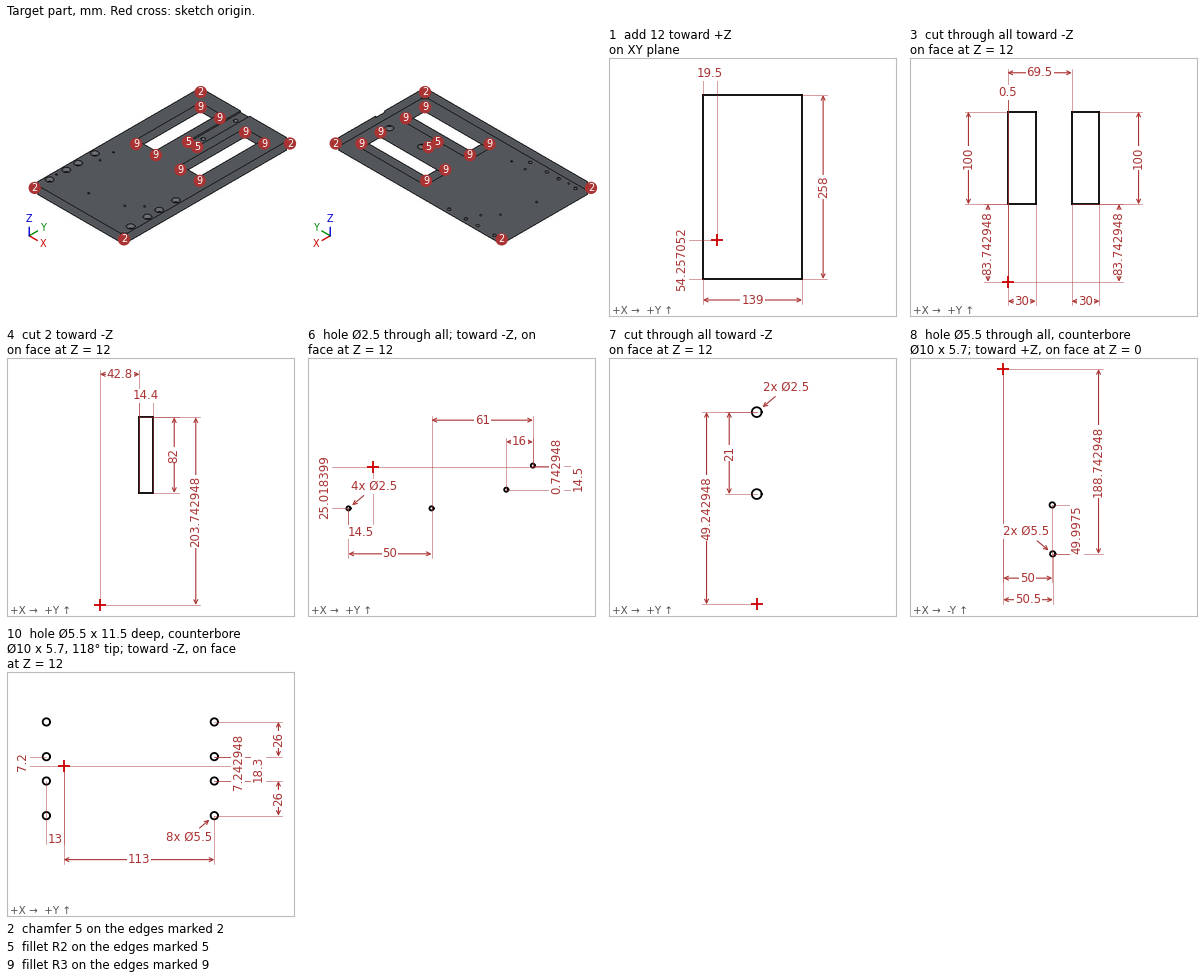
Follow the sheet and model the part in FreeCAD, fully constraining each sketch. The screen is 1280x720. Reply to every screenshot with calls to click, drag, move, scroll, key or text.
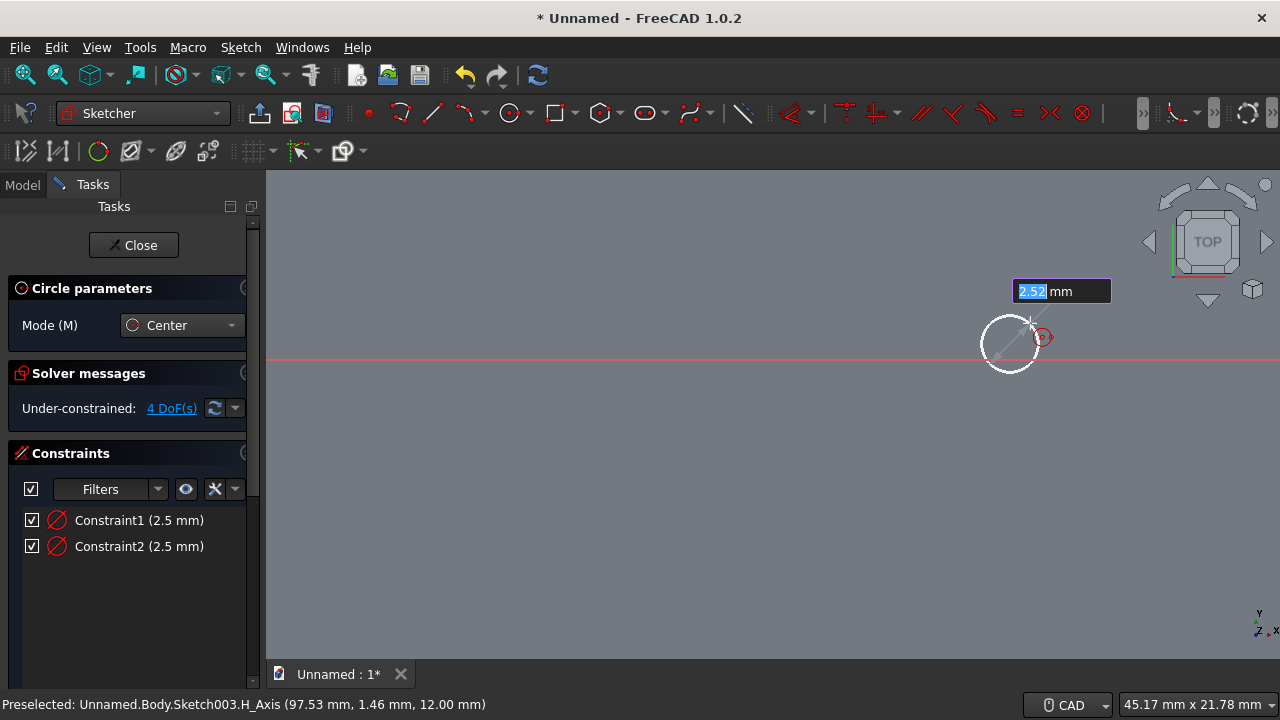
text(2.5)
key(Return)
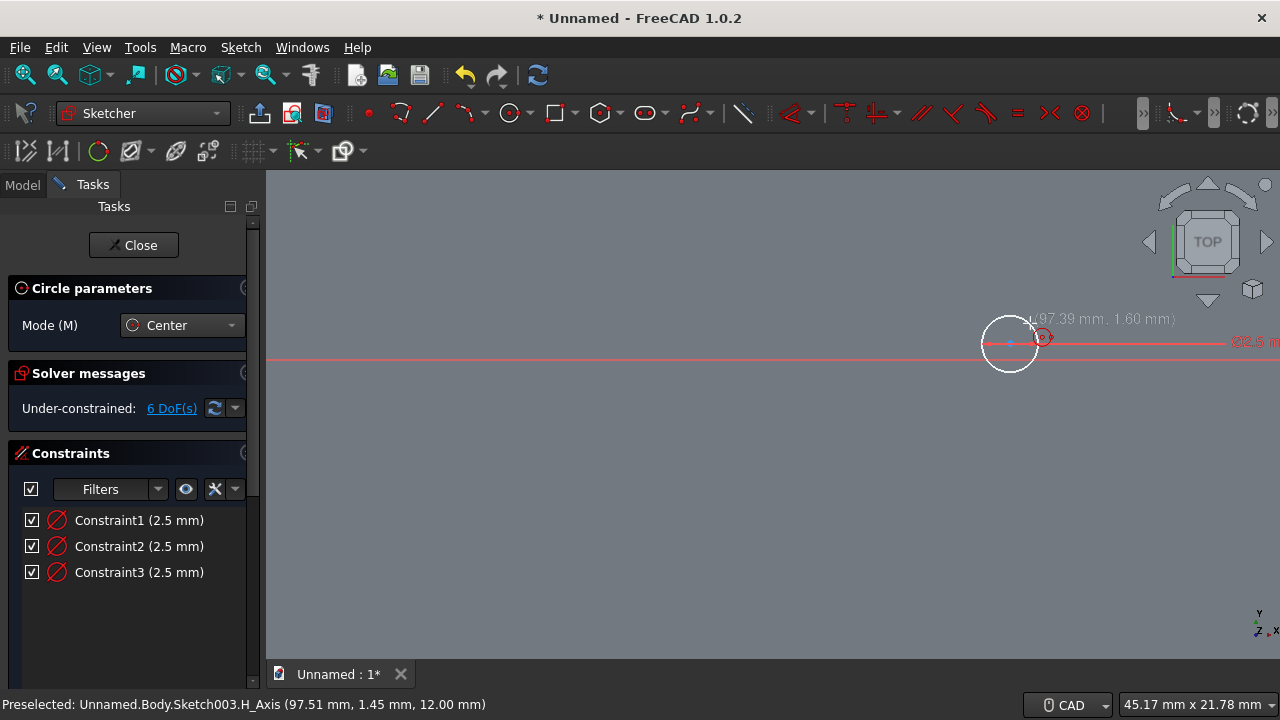
scroll(1012, 343, down, 7)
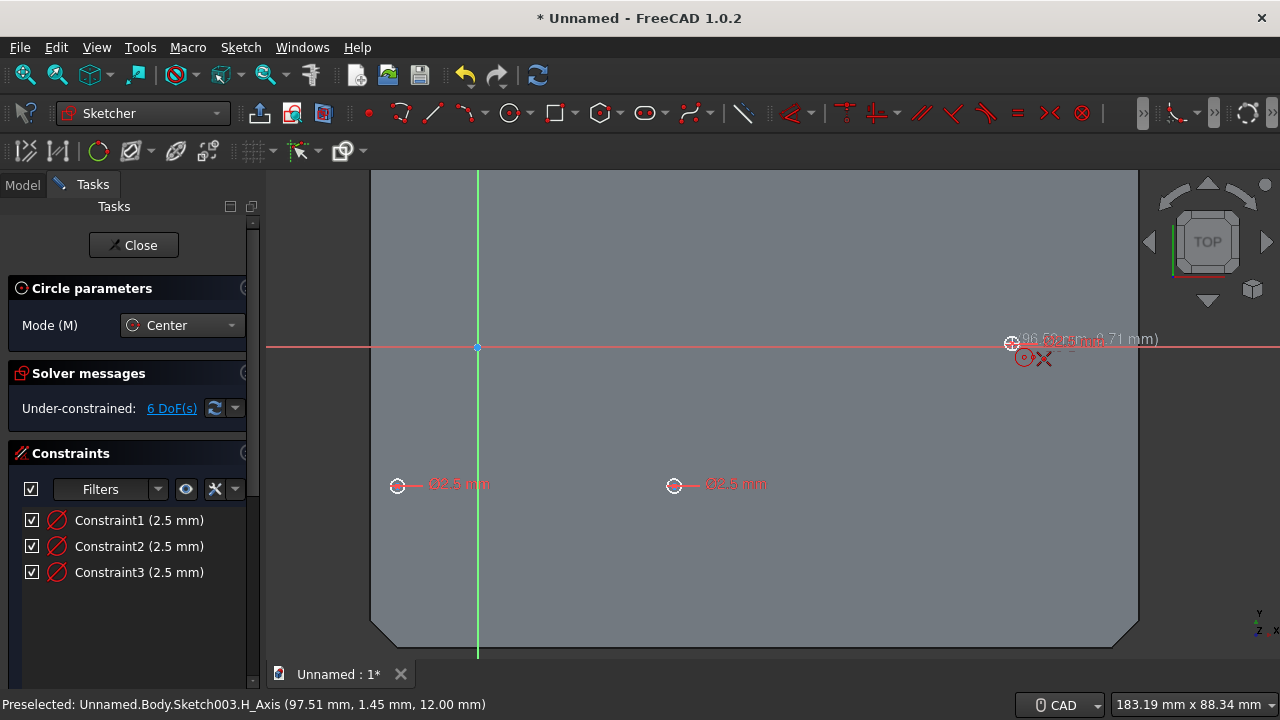
scroll(923, 424, up, 6)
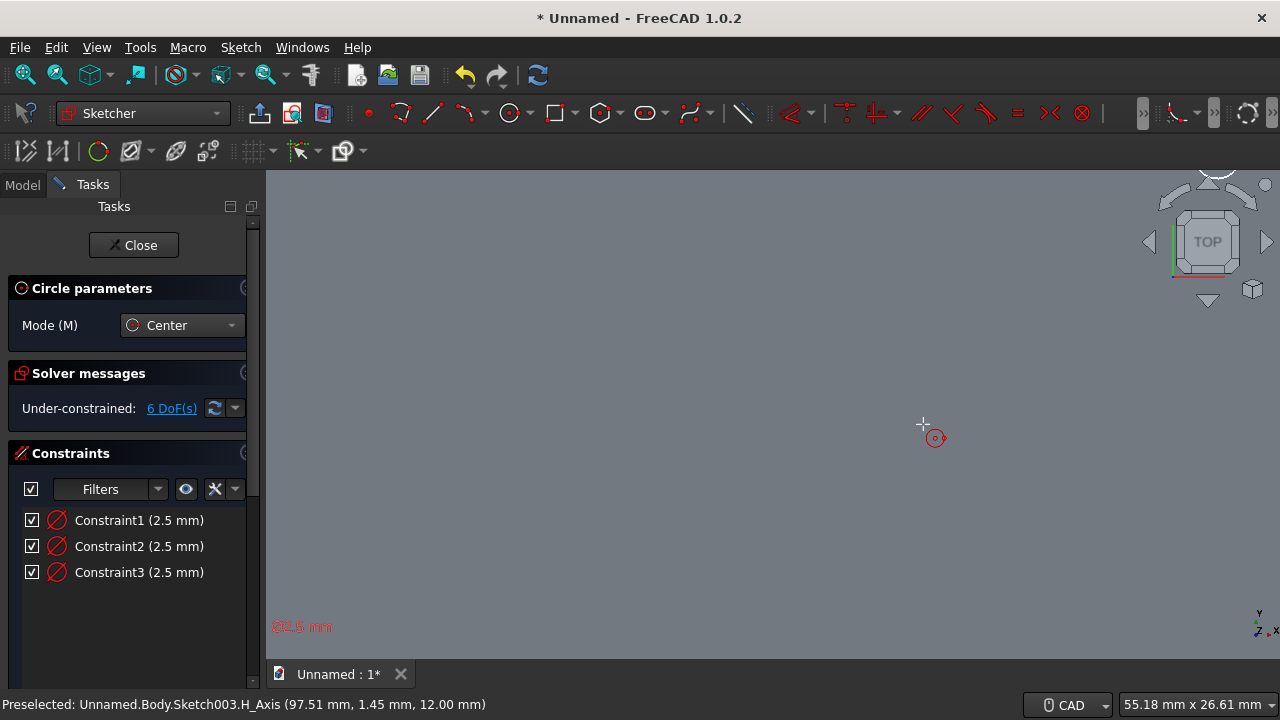
click(923, 421)
move(939, 405)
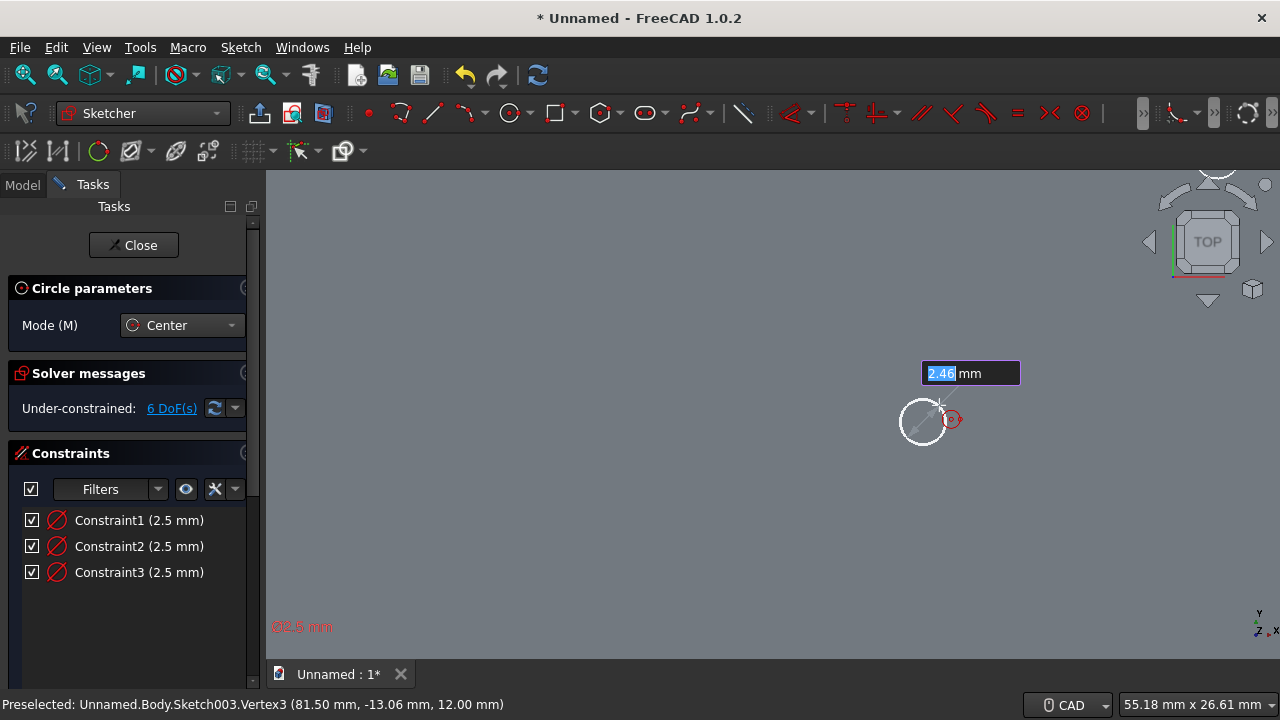
text(2.5)
key(Return)
key(Escape)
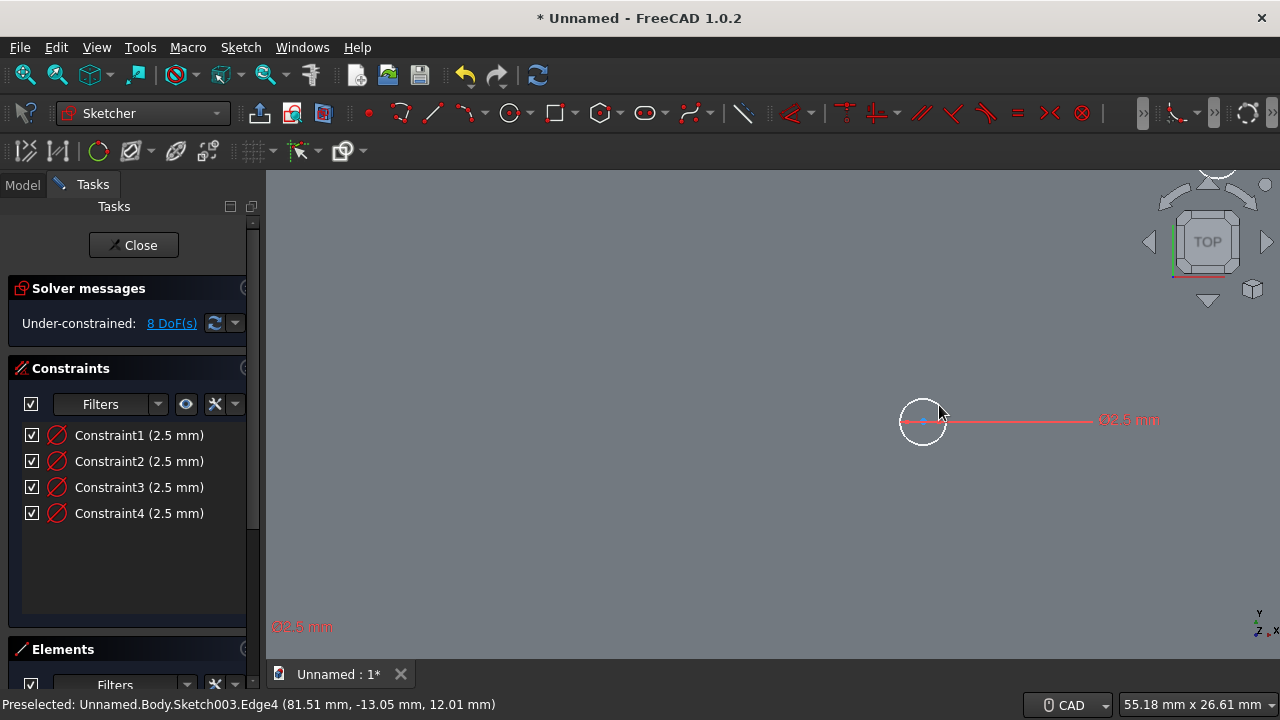
scroll(923, 424, down, 6)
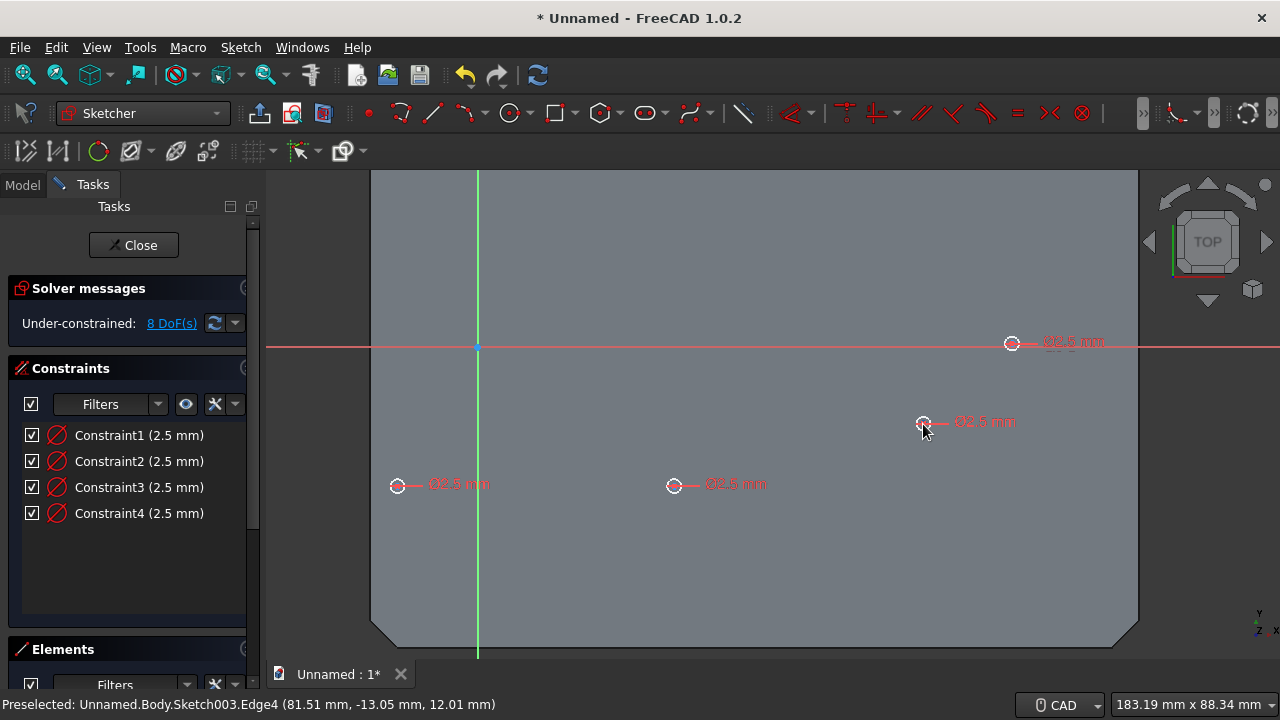
click(397, 486)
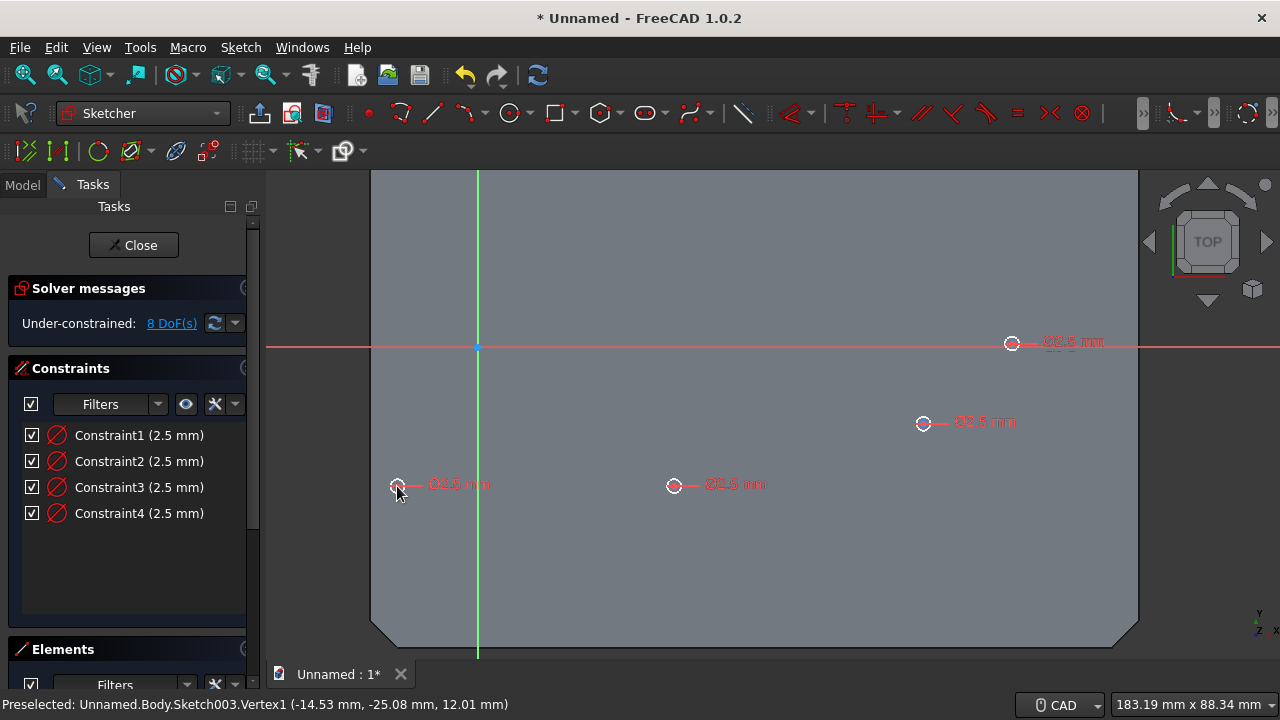
click(674, 486)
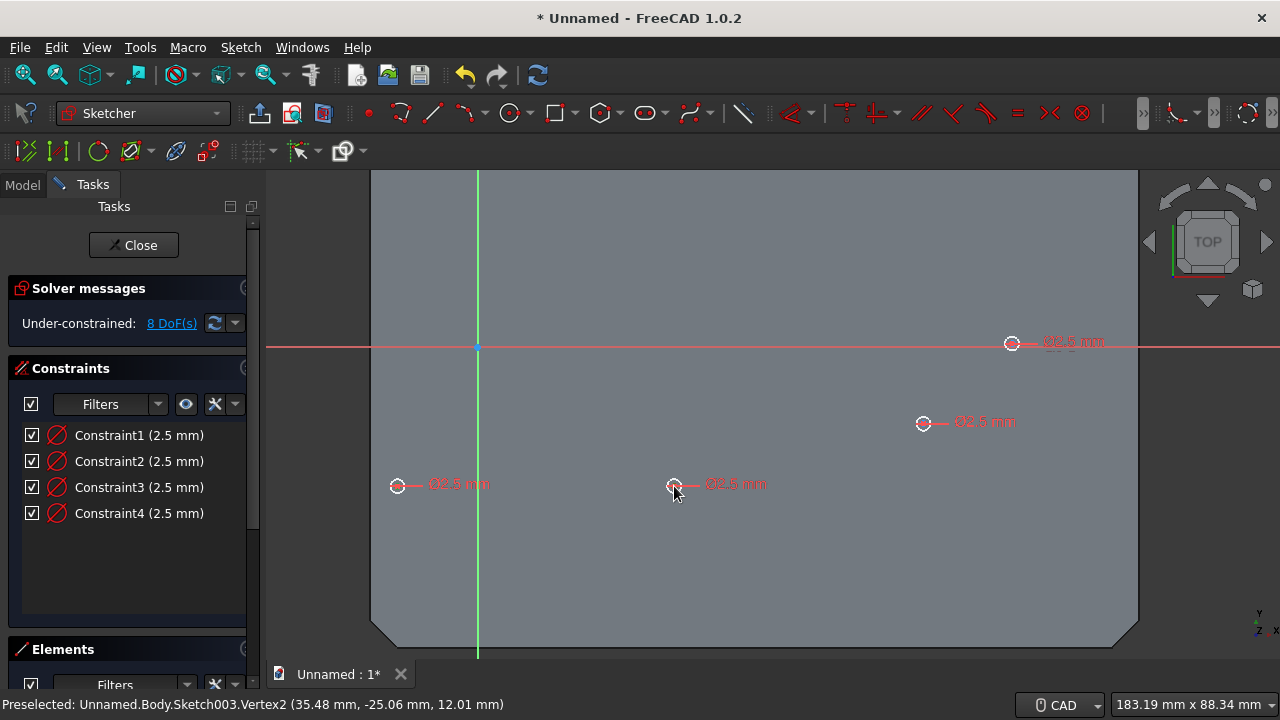
key(h)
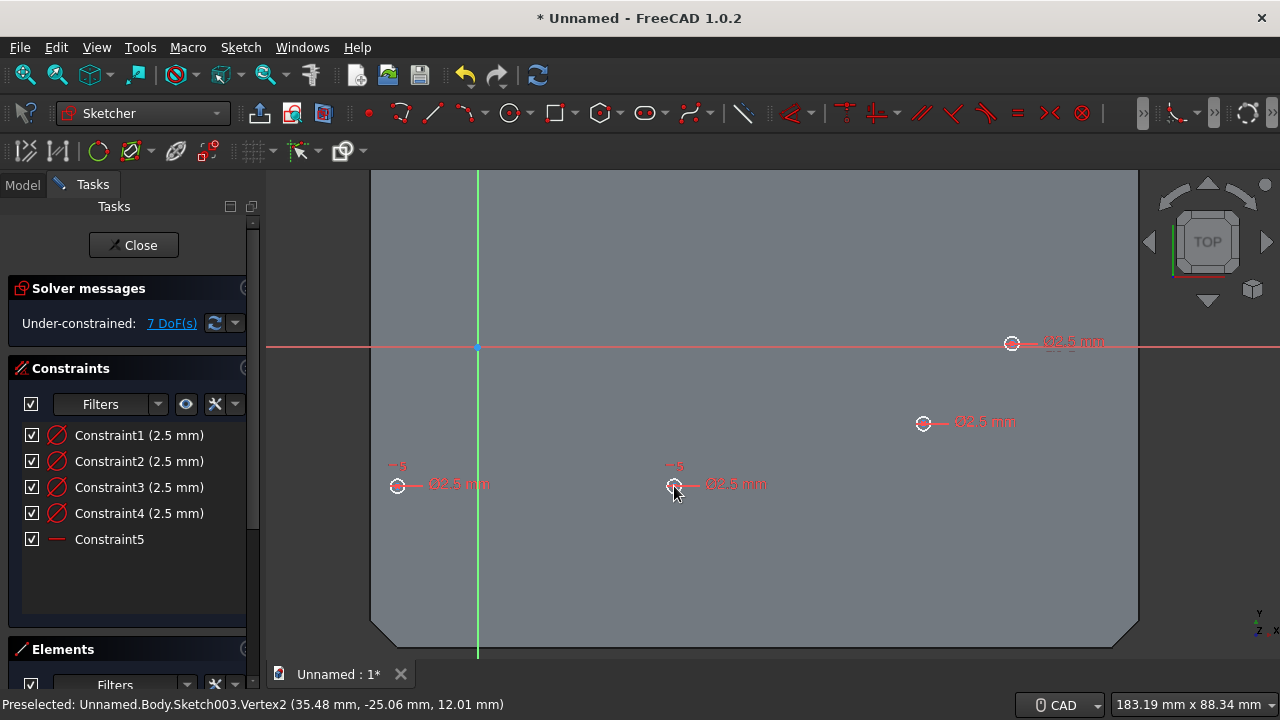
click(790, 114)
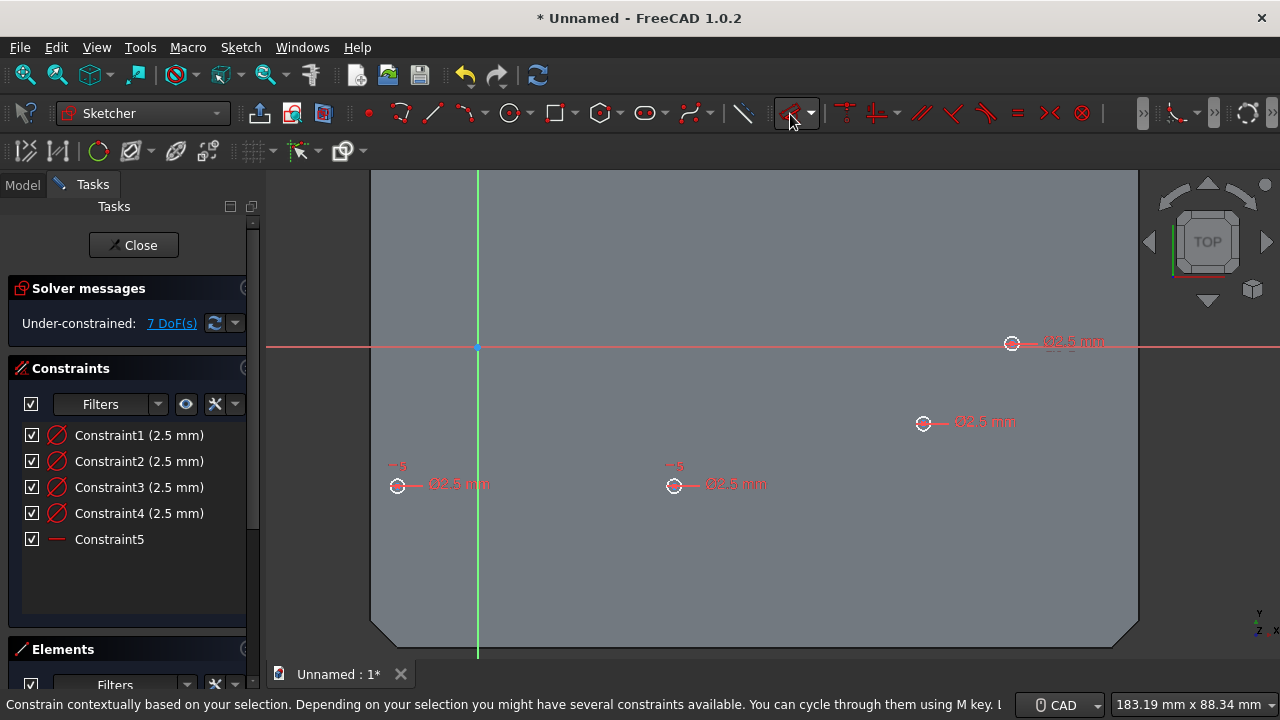
click(397, 486)